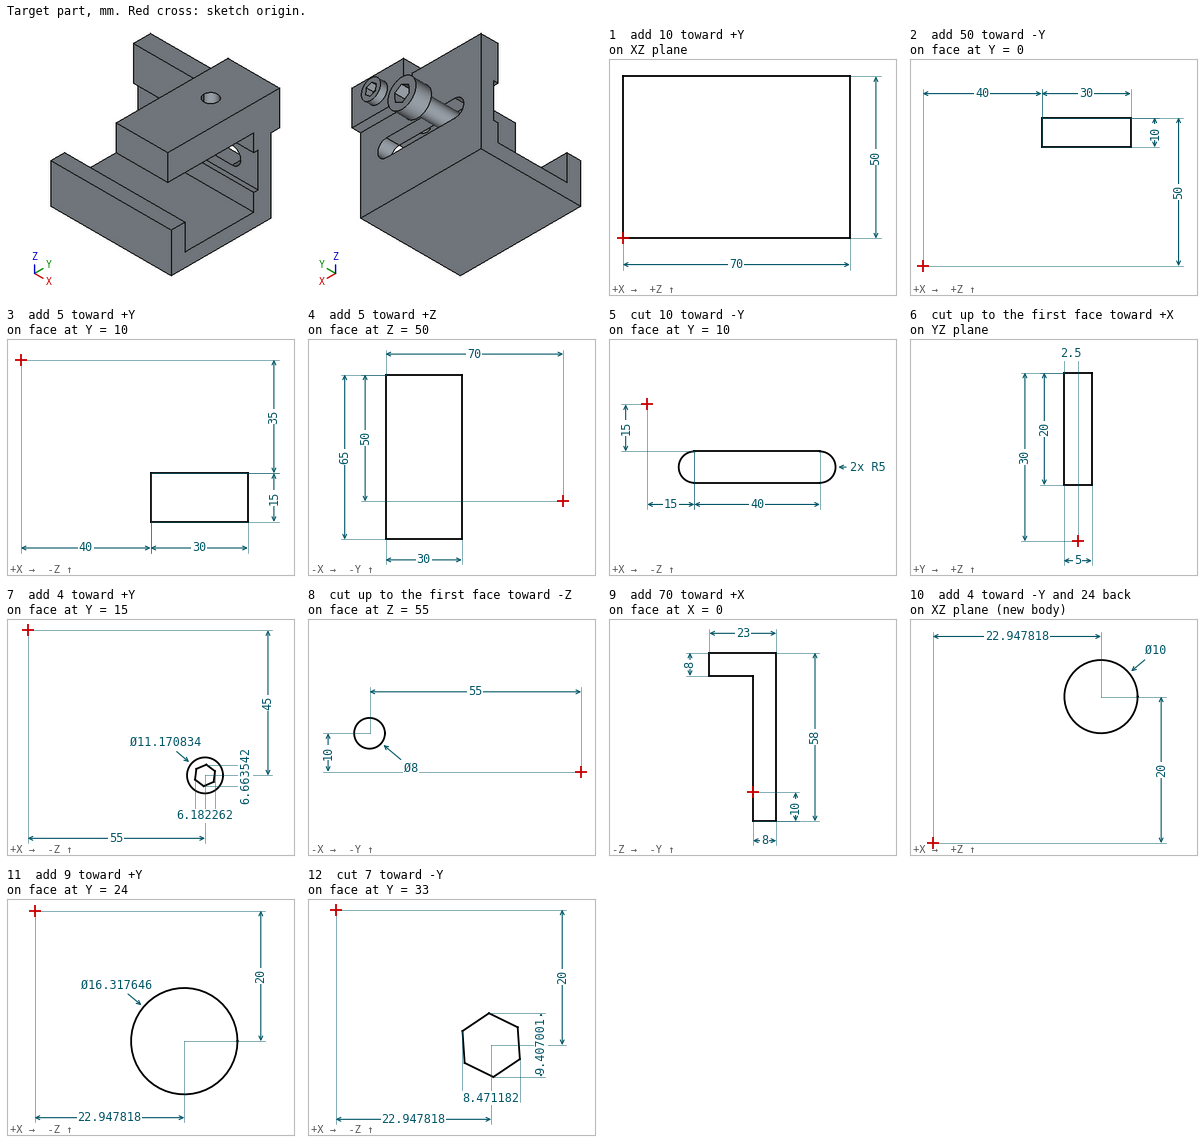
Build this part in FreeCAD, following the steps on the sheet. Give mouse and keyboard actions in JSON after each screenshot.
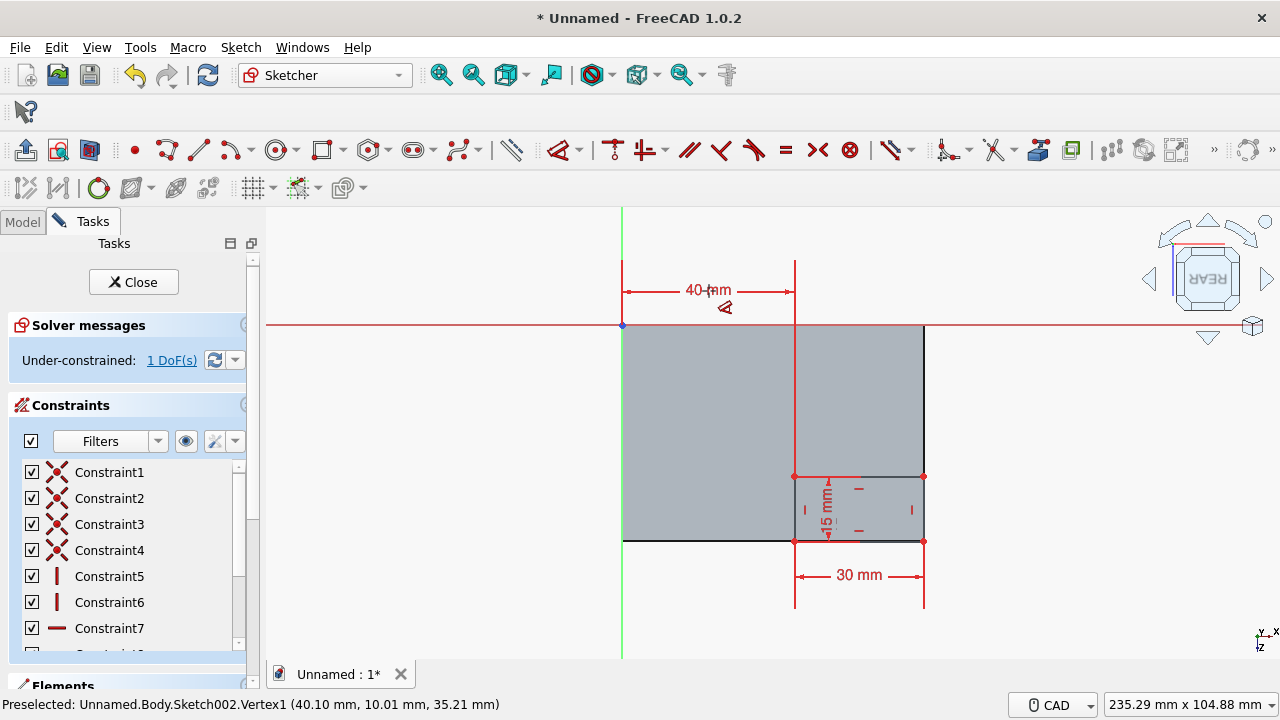
{"action": "left_click", "coordinate": [795, 477]}
{"action": "left_click", "coordinate": [588, 401]}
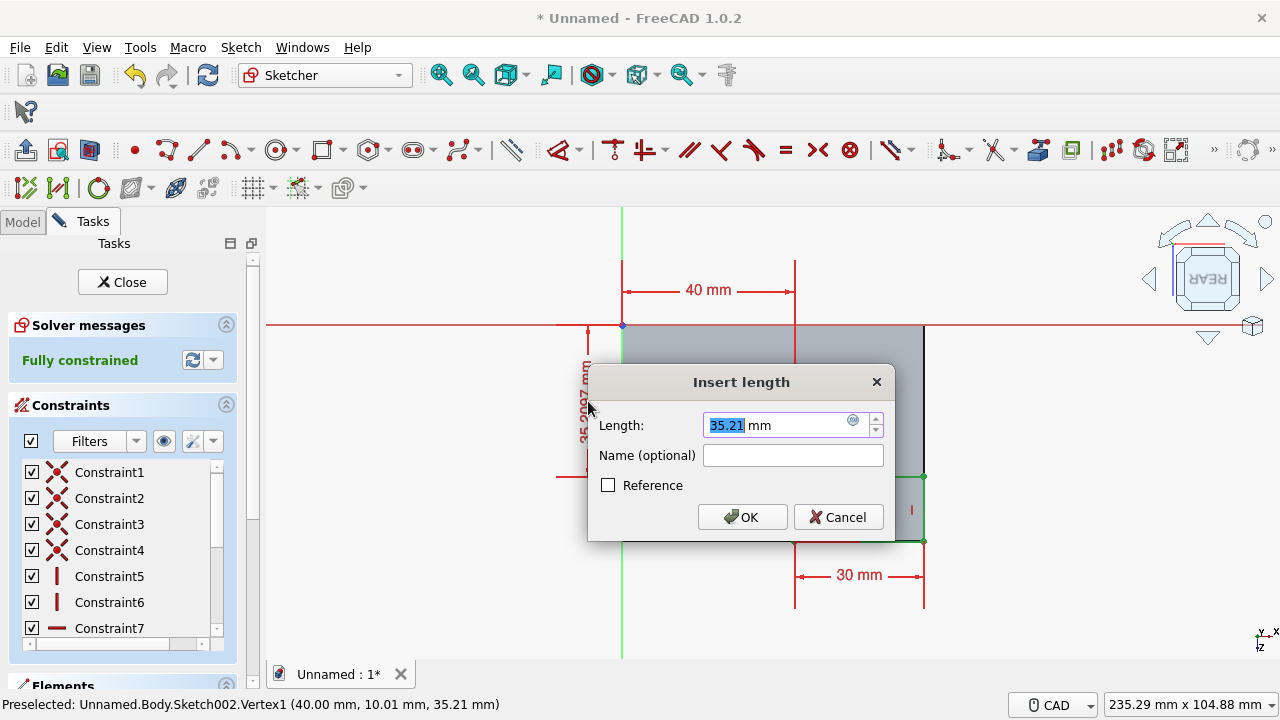
{"action": "type", "text": "35"}
{"action": "key", "text": "Return"}
{"action": "key", "text": "Escape"}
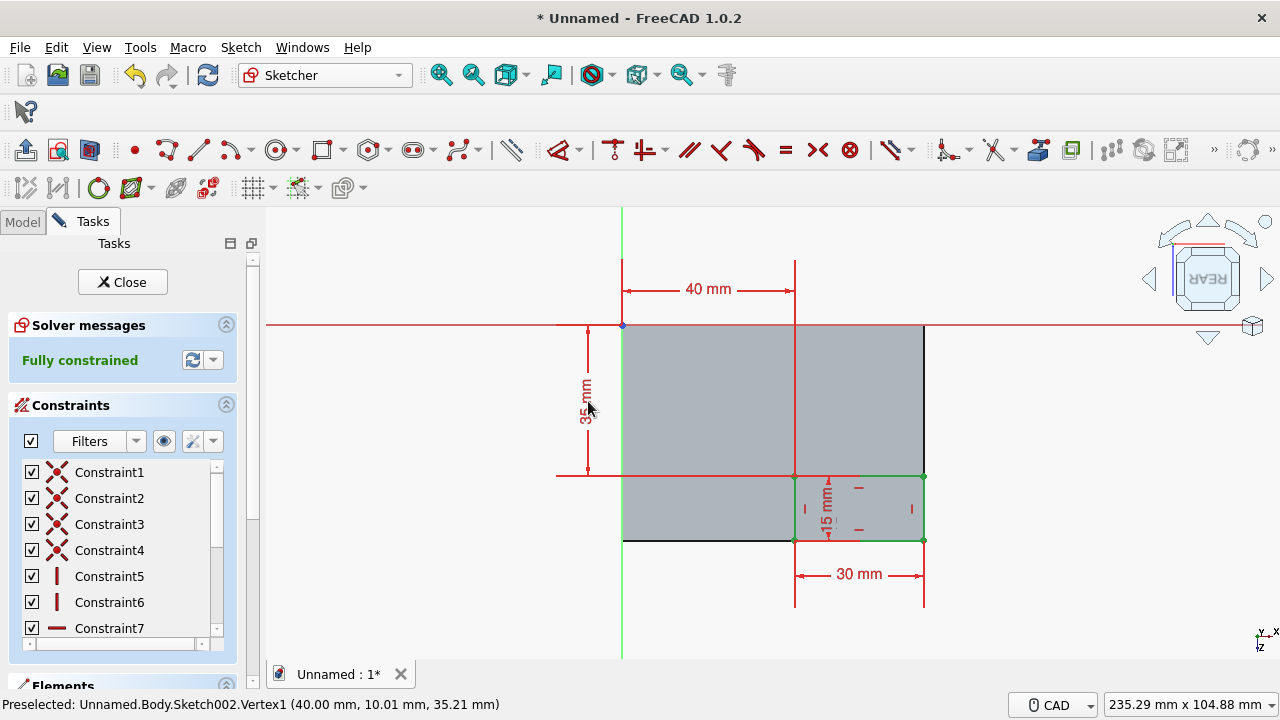
{"action": "left_click", "coordinate": [123, 282]}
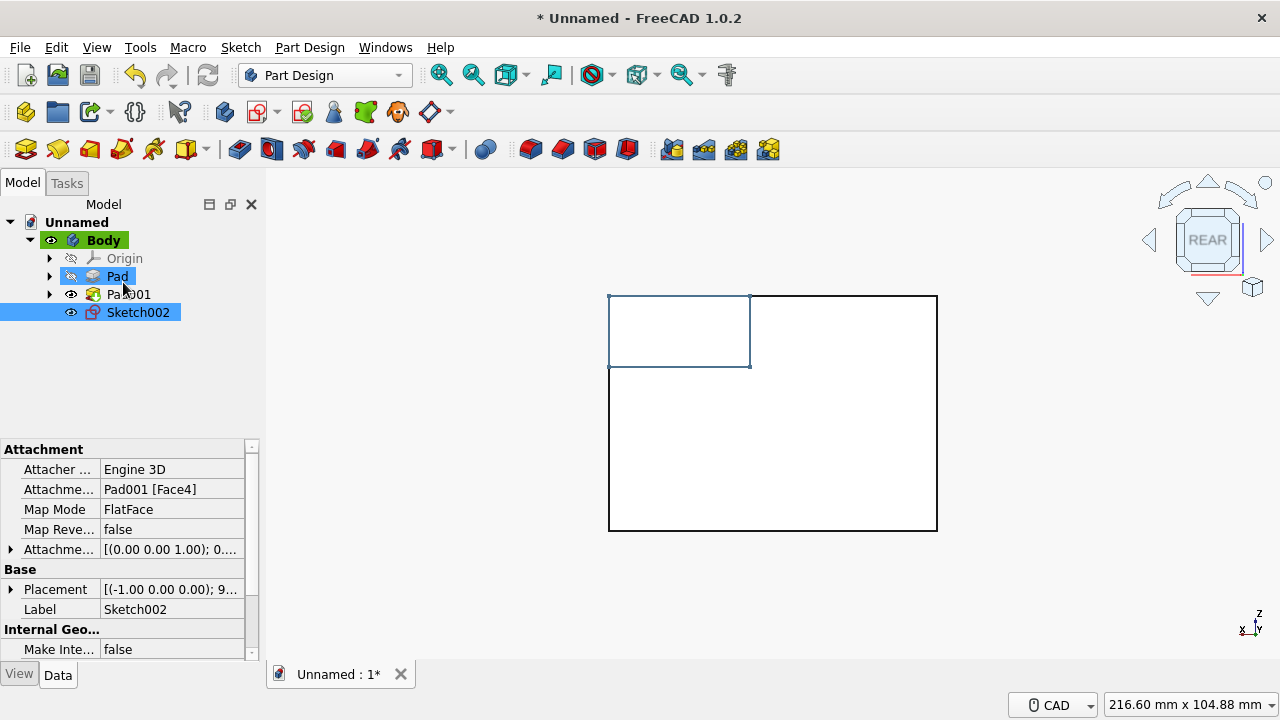
{"action": "left_click", "coordinate": [26, 150]}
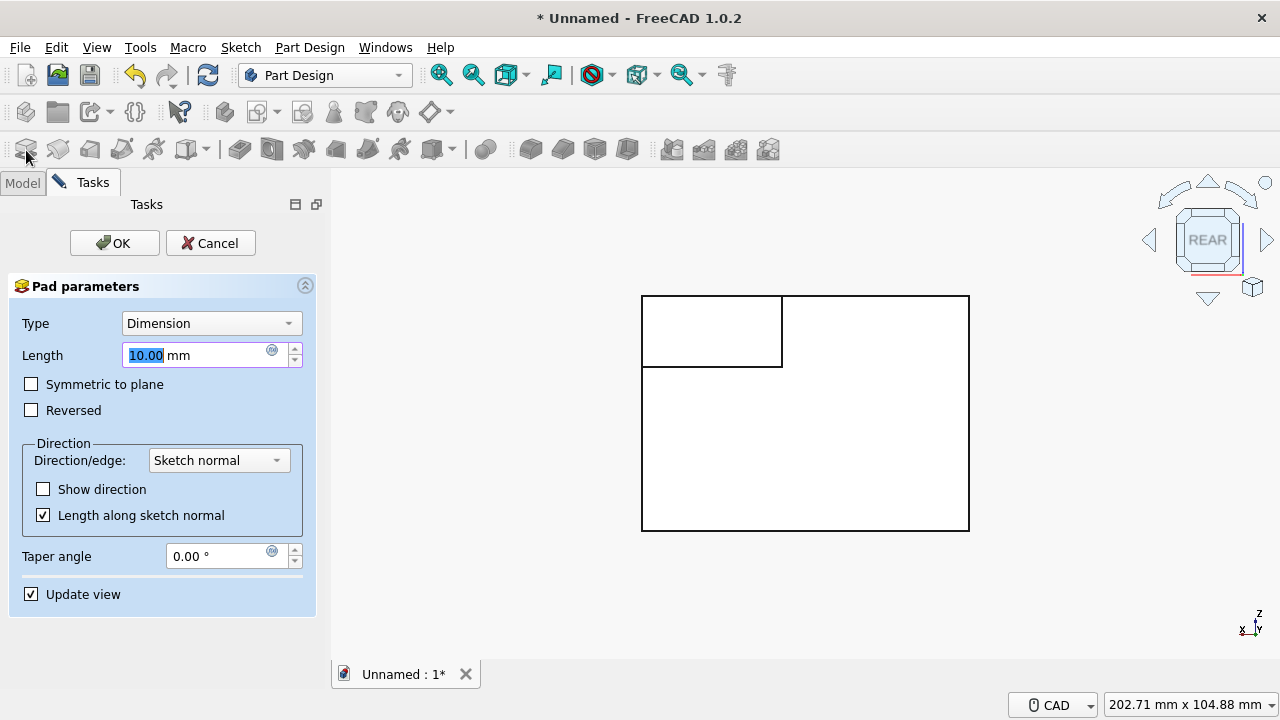
{"action": "type", "text": "5"}
{"action": "key", "text": "Tab"}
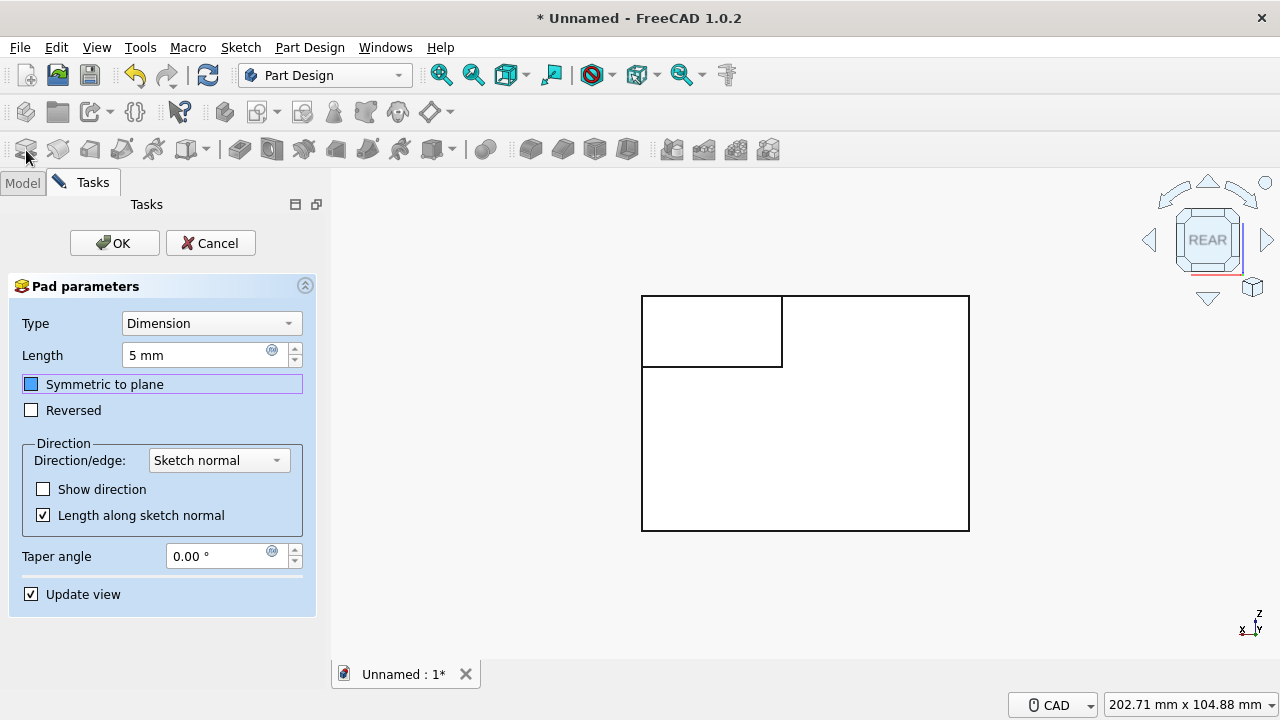
{"action": "left_click", "coordinate": [115, 243]}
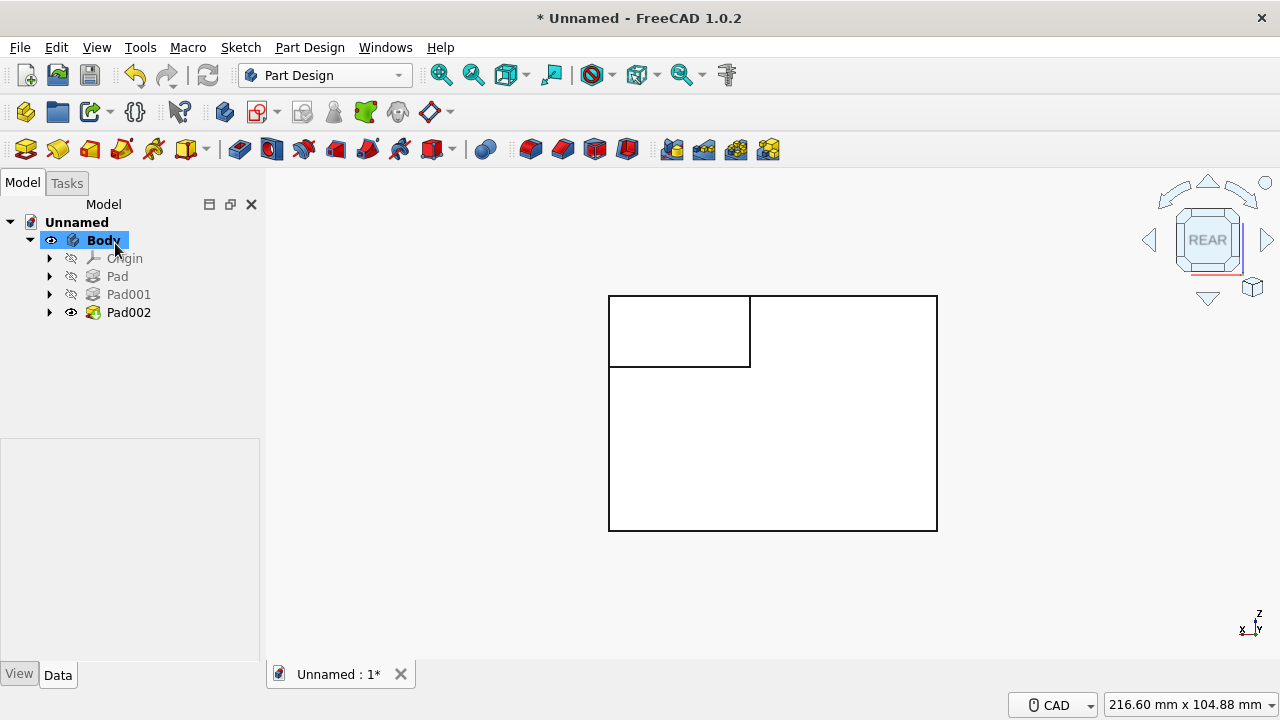
{"action": "key", "text": "0"}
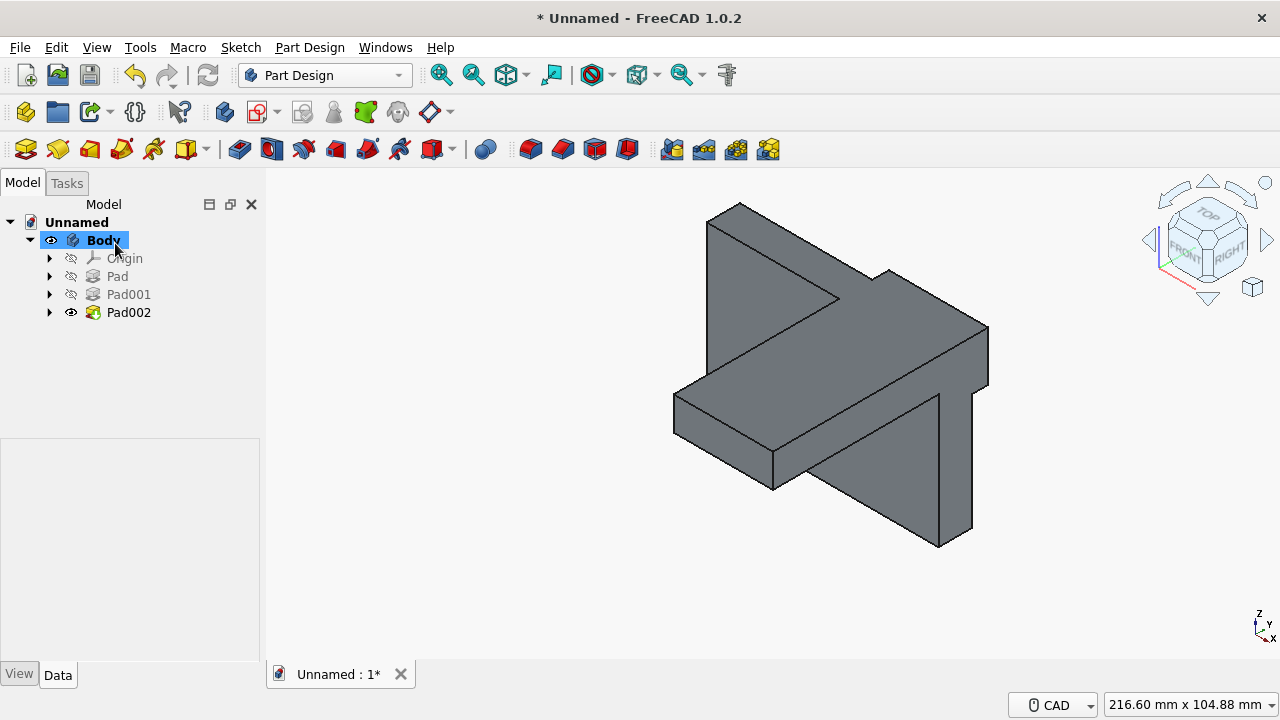
{"action": "left_click", "coordinate": [862, 342]}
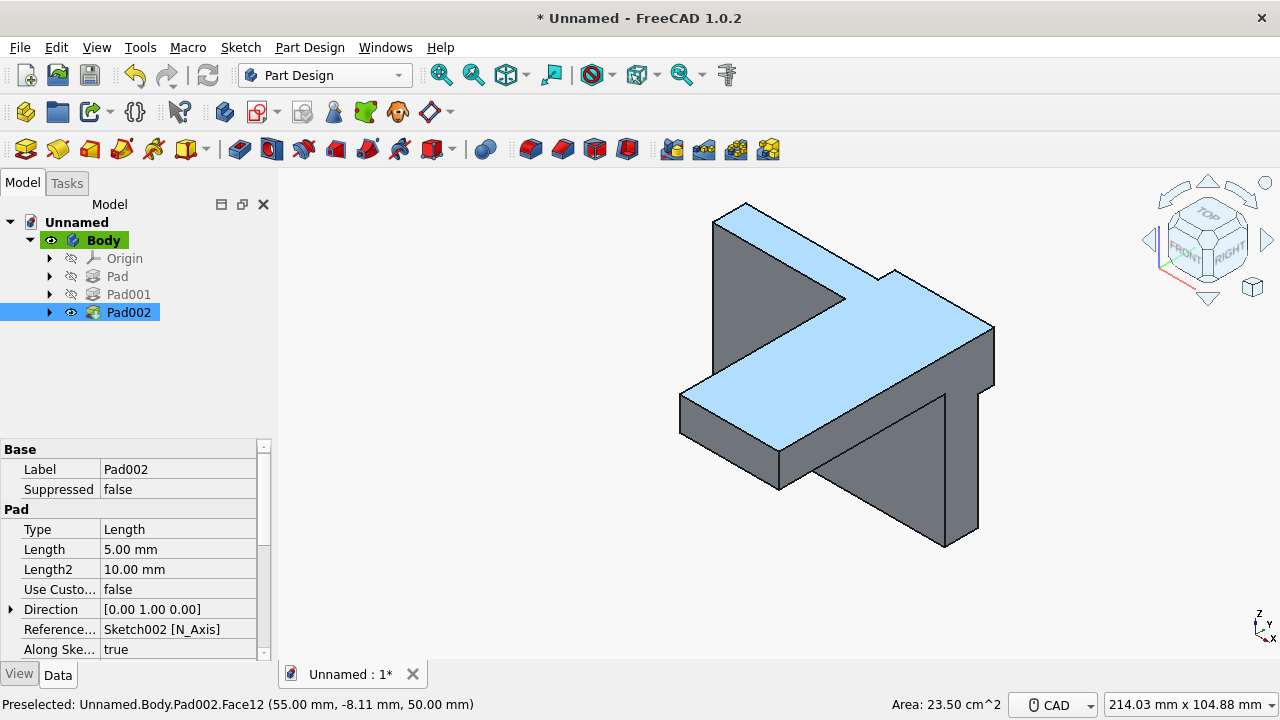
{"action": "left_click", "coordinate": [258, 112]}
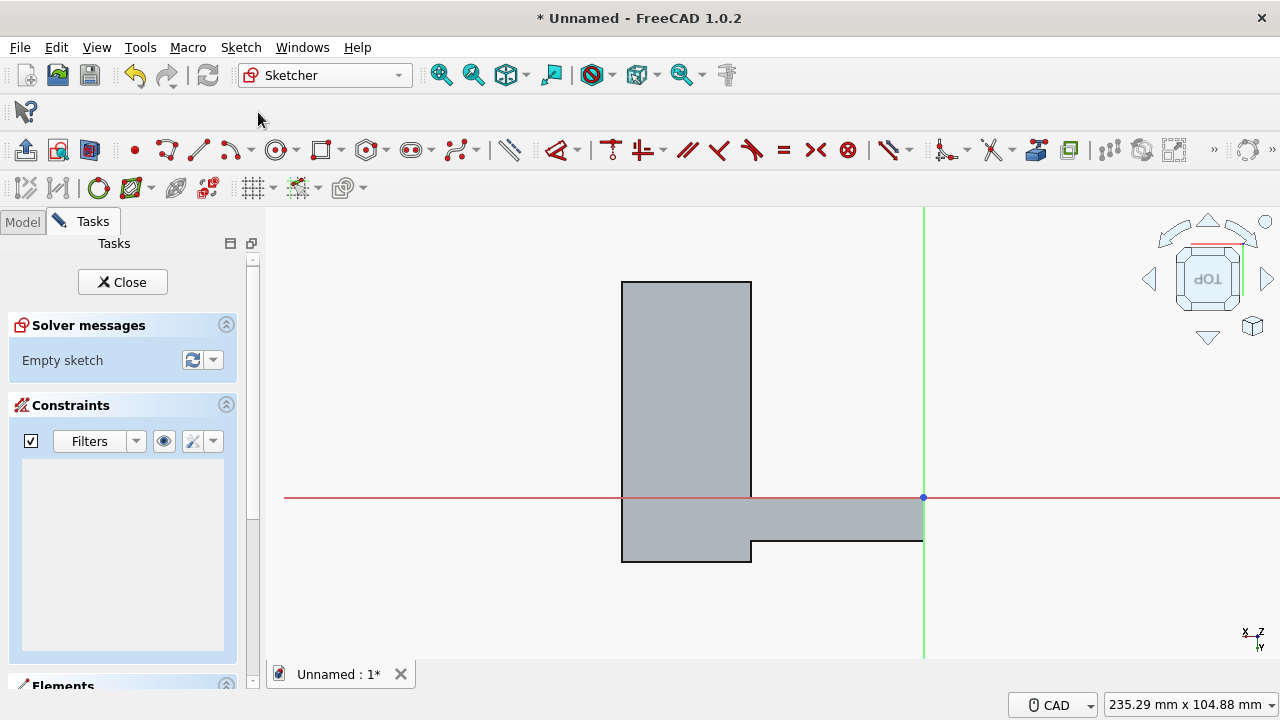
{"action": "left_click", "coordinate": [322, 150]}